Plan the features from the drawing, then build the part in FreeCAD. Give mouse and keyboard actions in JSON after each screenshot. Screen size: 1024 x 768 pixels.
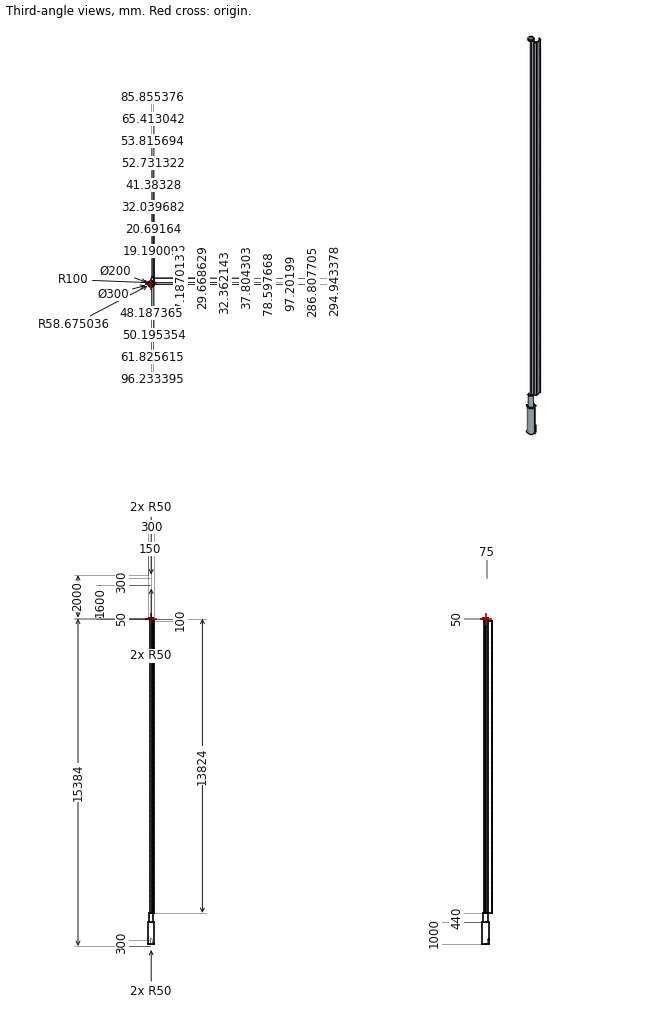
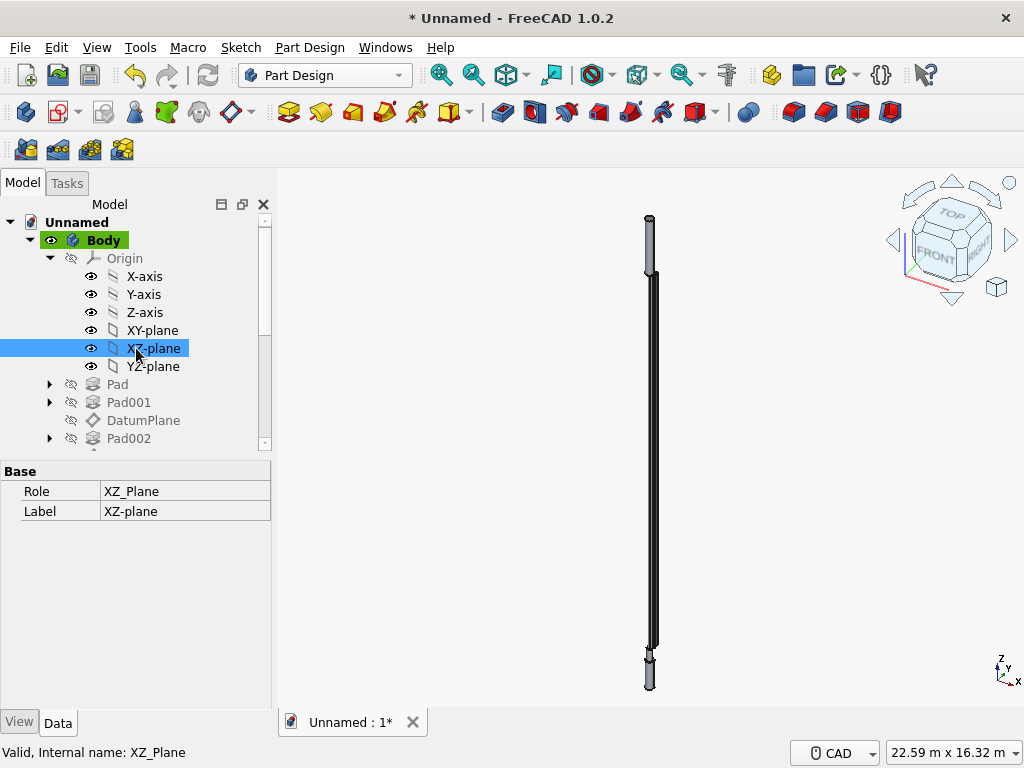
{"action": "left_click", "coordinate": [232, 112]}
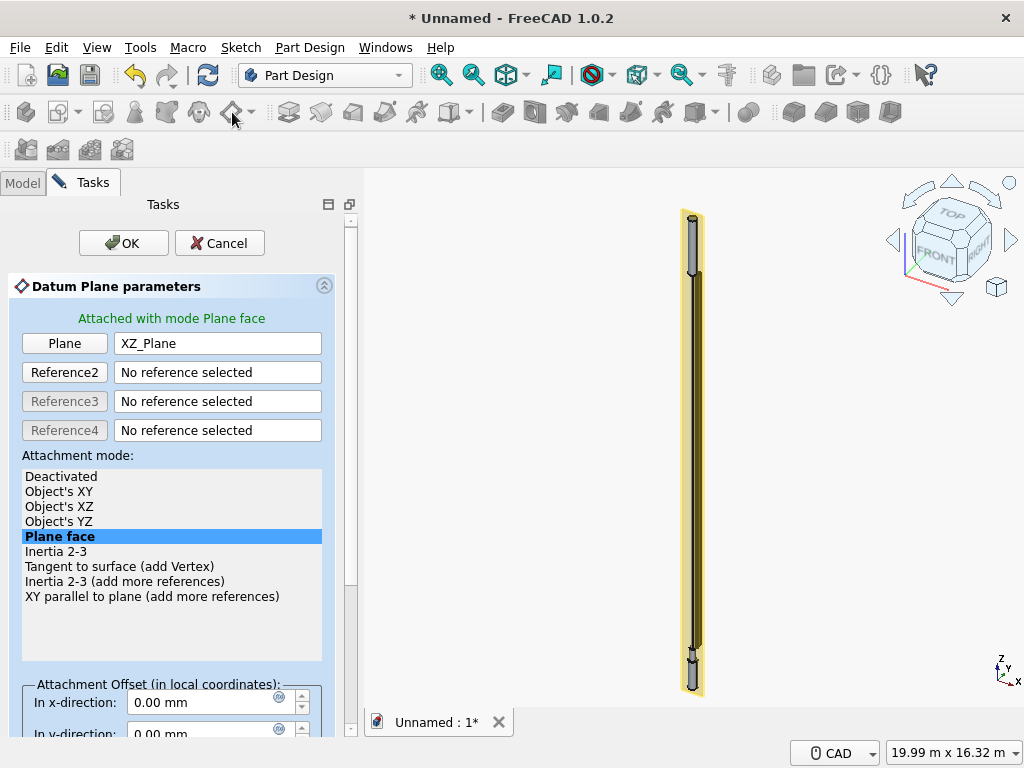
{"action": "scroll", "coordinate": [351, 475], "scroll_direction": "down", "scroll_amount": 2}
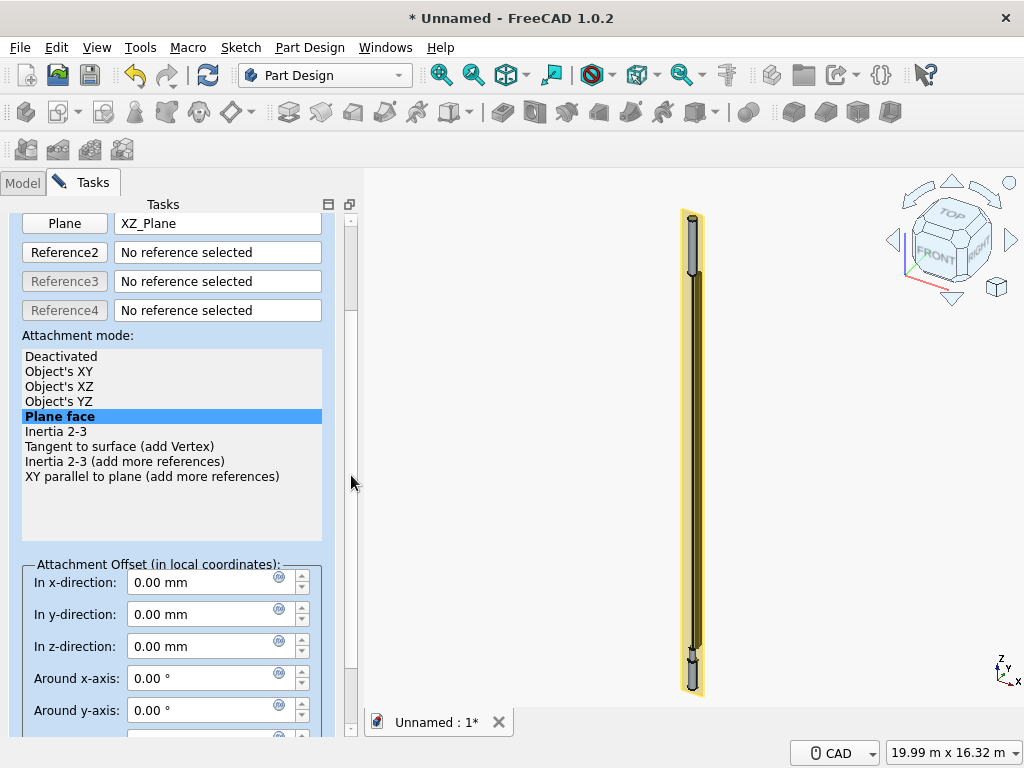
{"action": "triple_click", "coordinate": [210, 646]}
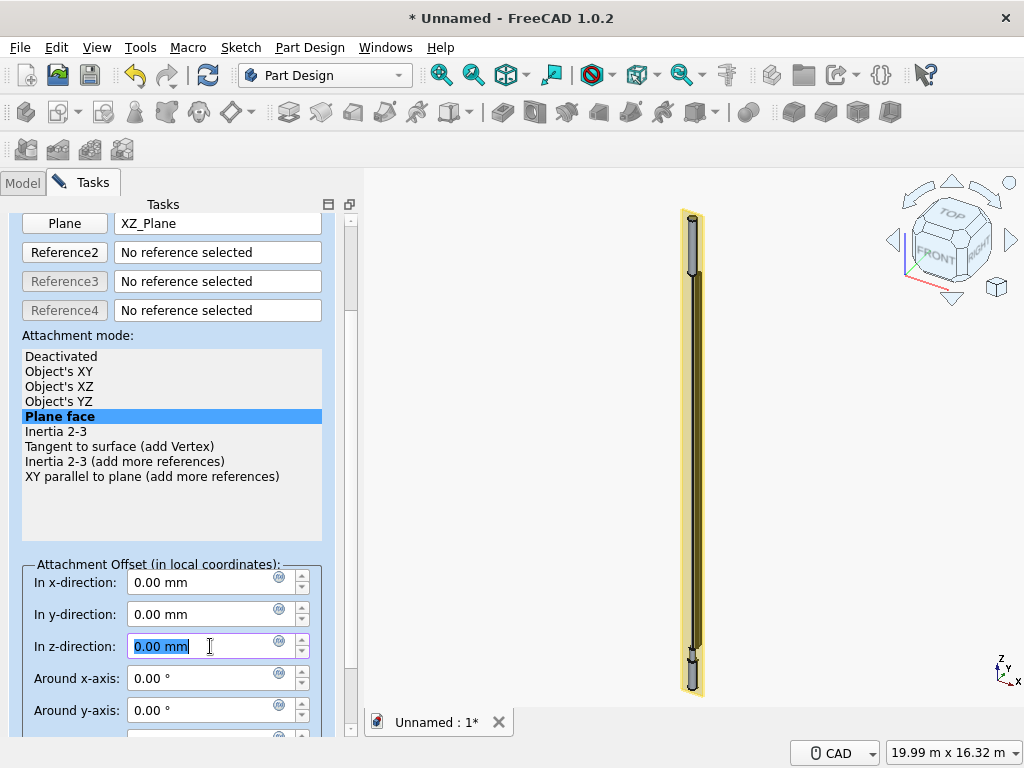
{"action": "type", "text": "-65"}
{"action": "key", "text": "Tab"}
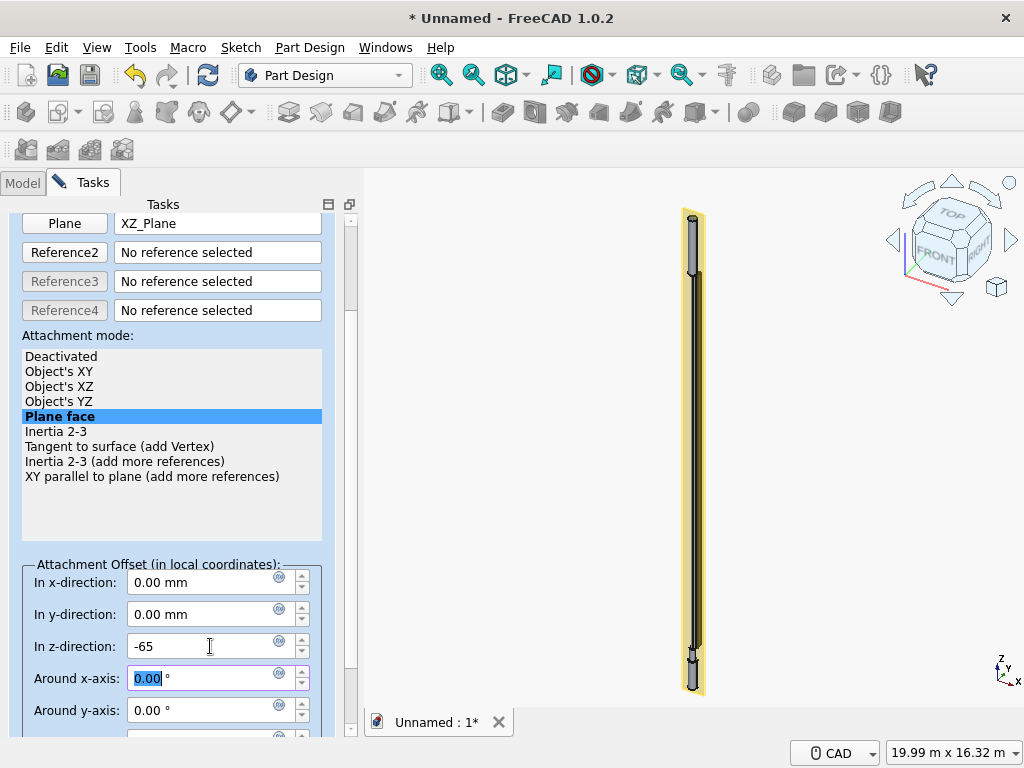
{"action": "scroll", "coordinate": [351, 475], "scroll_direction": "up", "scroll_amount": 3}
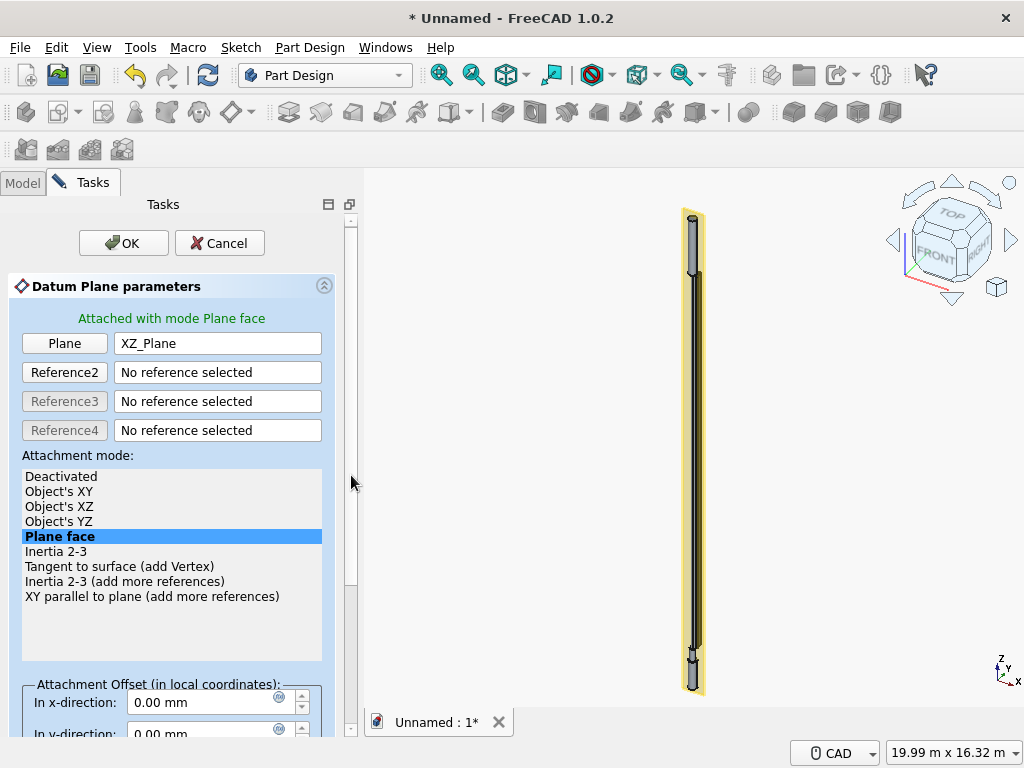
{"action": "left_click", "coordinate": [124, 243]}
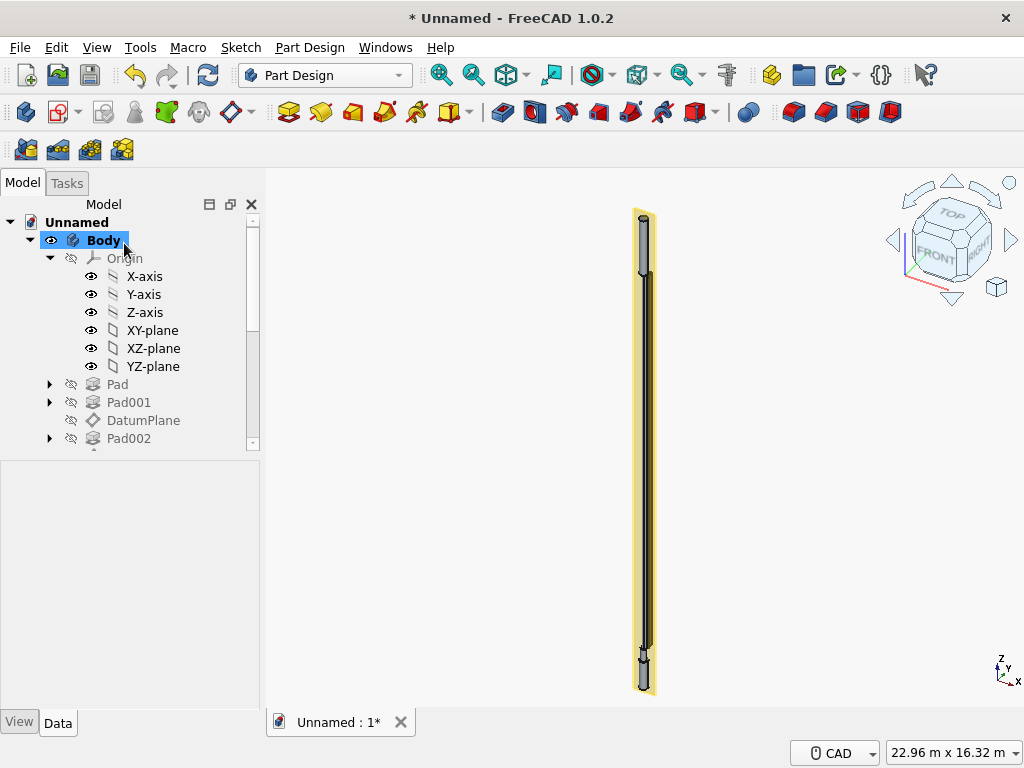
{"action": "scroll", "coordinate": [100, 326], "scroll_direction": "down", "scroll_amount": 3}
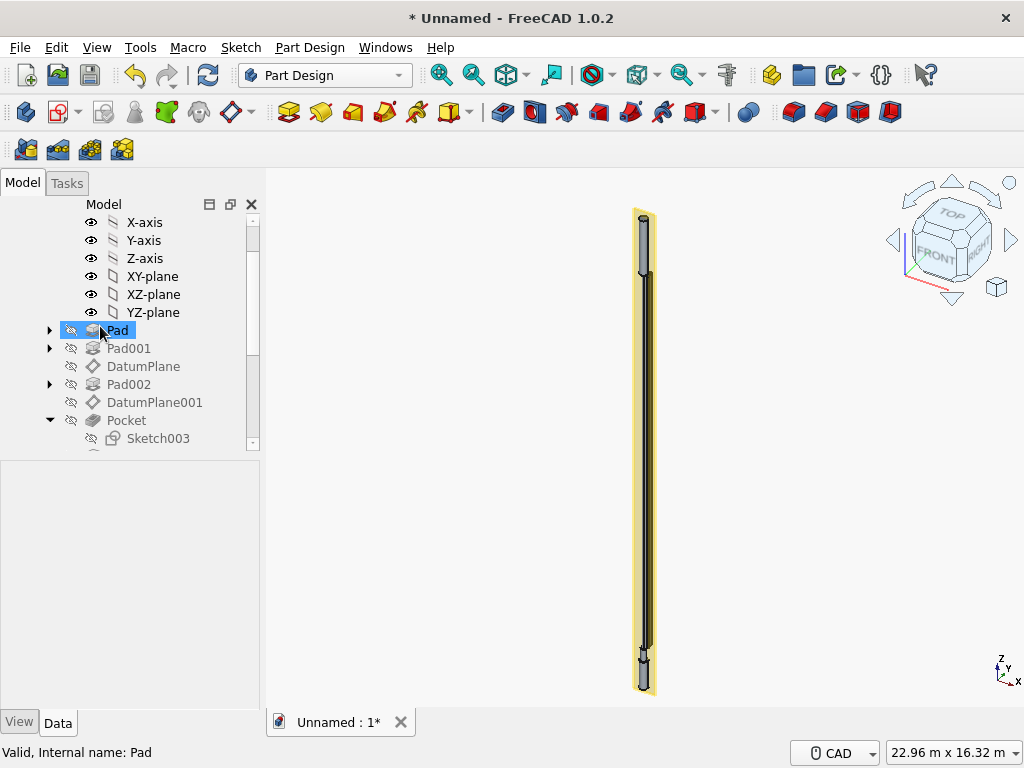
{"action": "scroll", "coordinate": [140, 326], "scroll_direction": "up", "scroll_amount": 15}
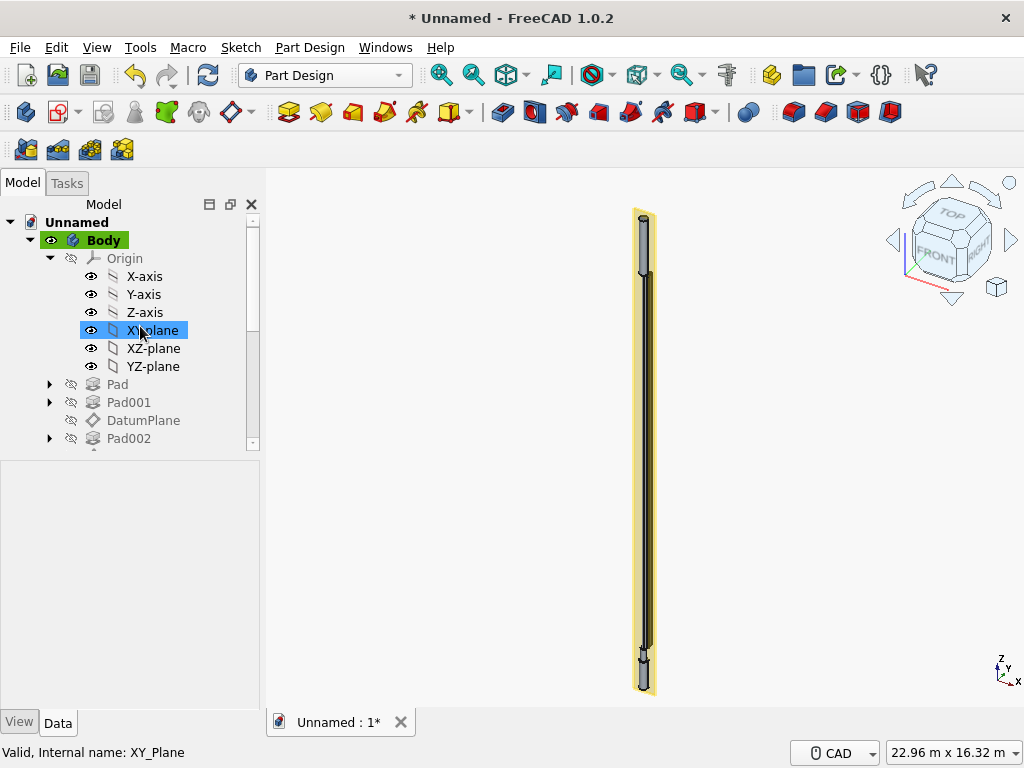
{"action": "scroll", "coordinate": [100, 326], "scroll_direction": "down", "scroll_amount": 6}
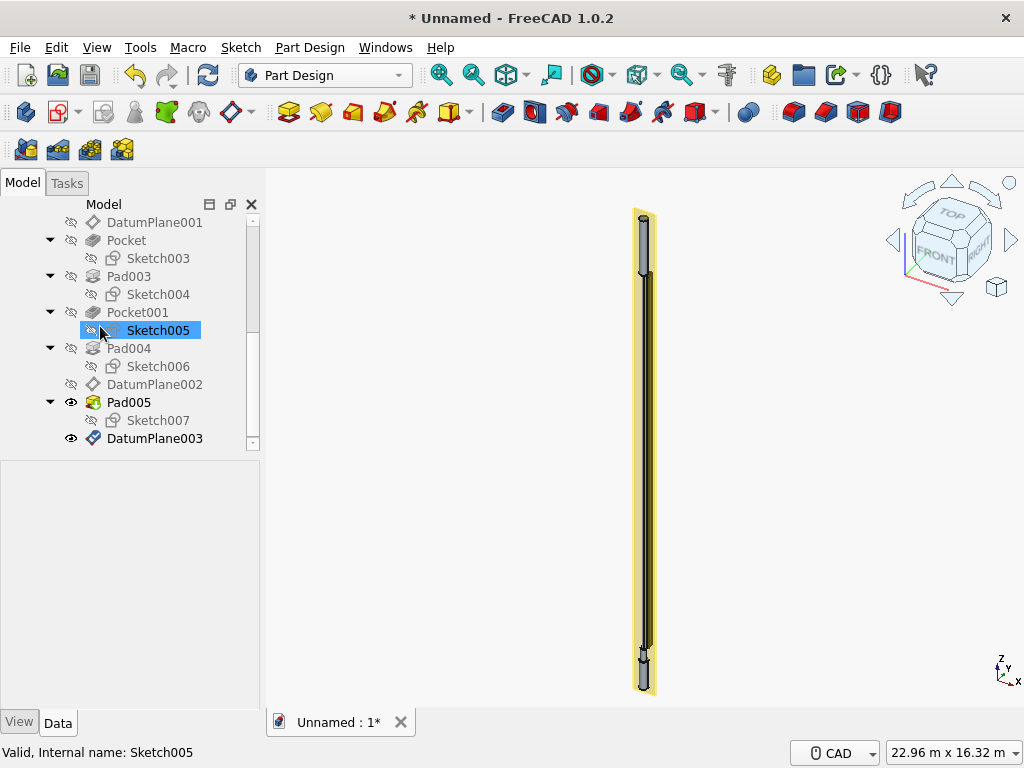
{"action": "left_click", "coordinate": [116, 438]}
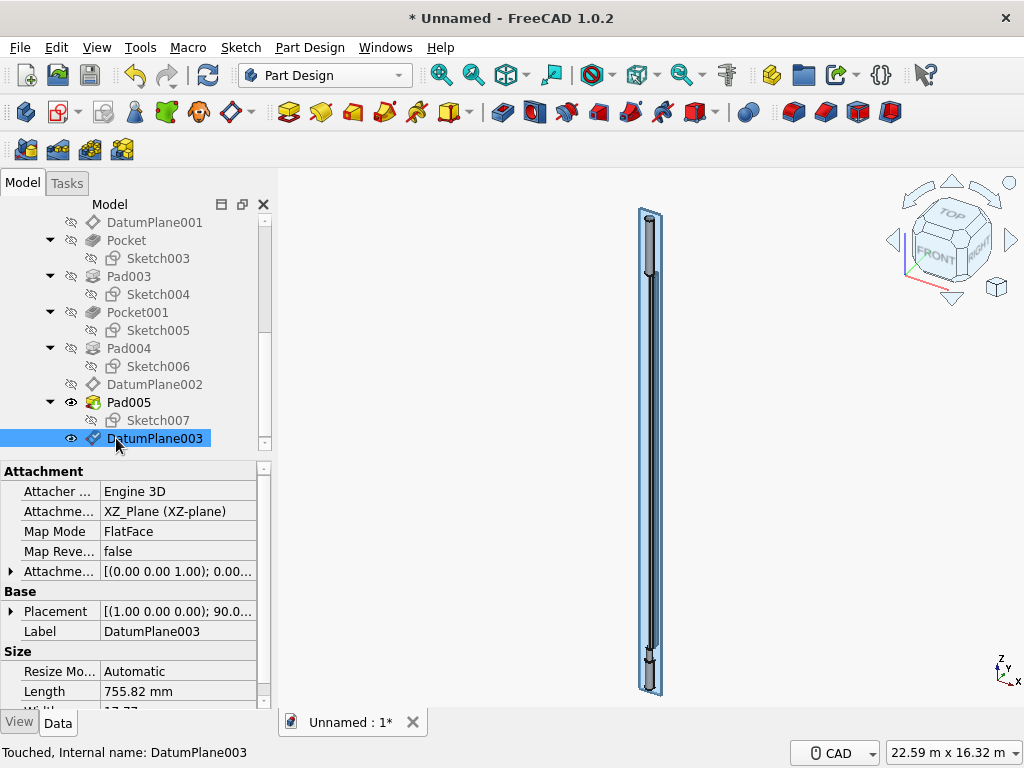
{"action": "left_click", "coordinate": [58, 112]}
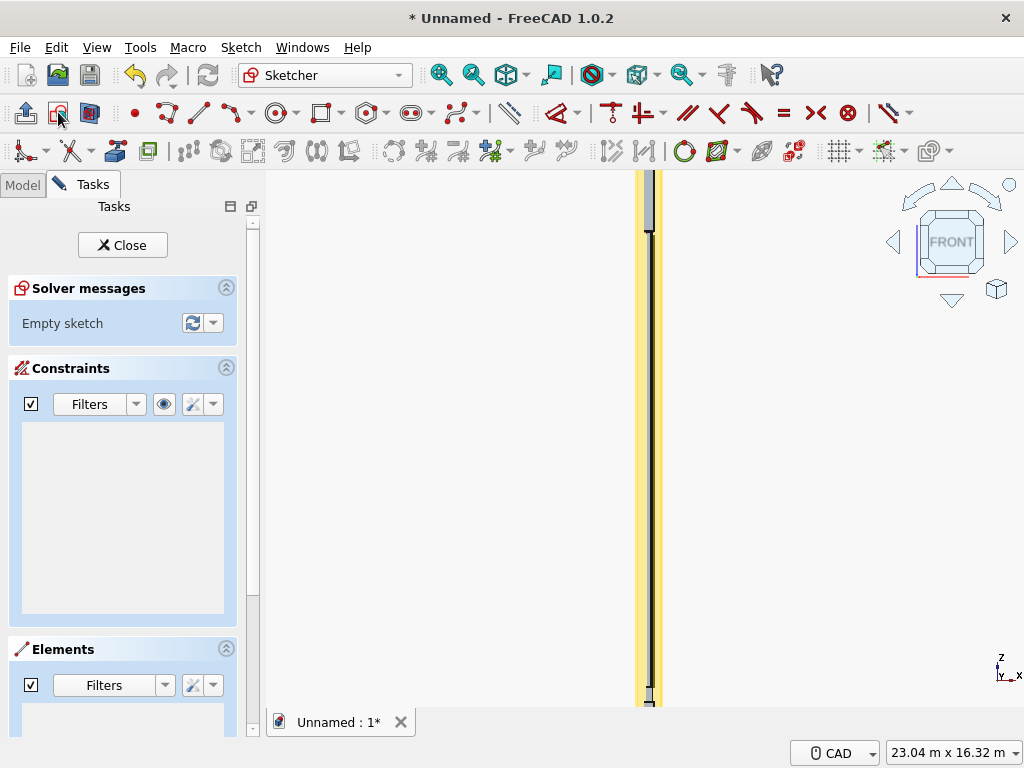
{"action": "left_click", "coordinate": [90, 114]}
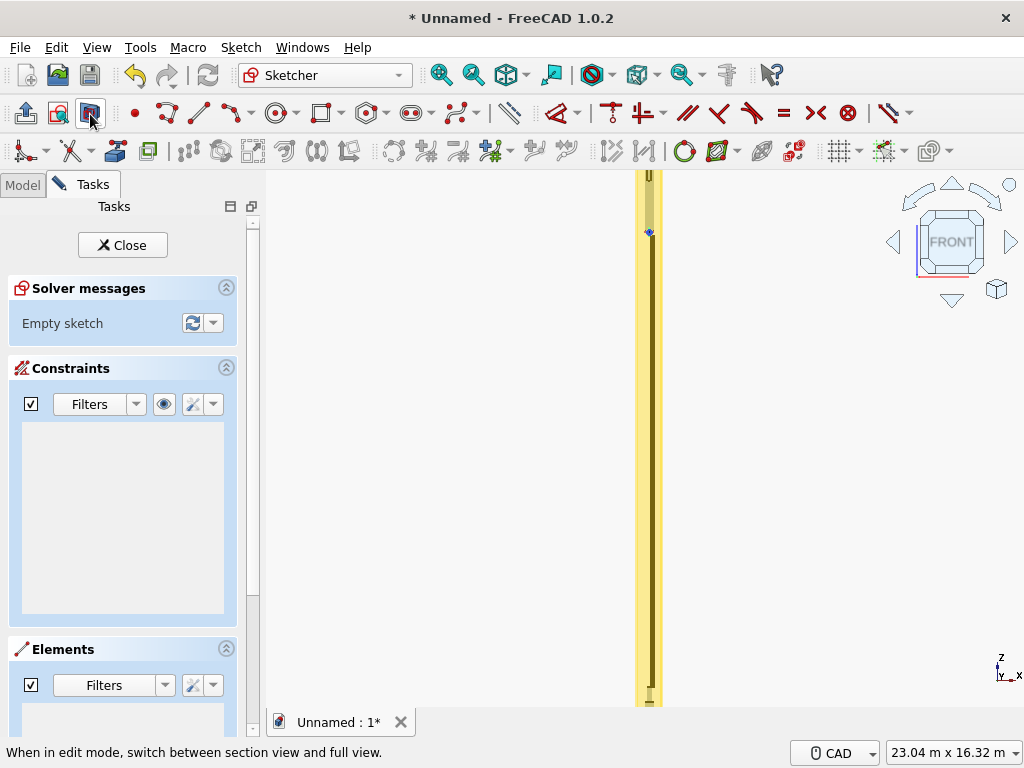
{"action": "scroll", "coordinate": [576, 438], "scroll_direction": "down", "scroll_amount": 5}